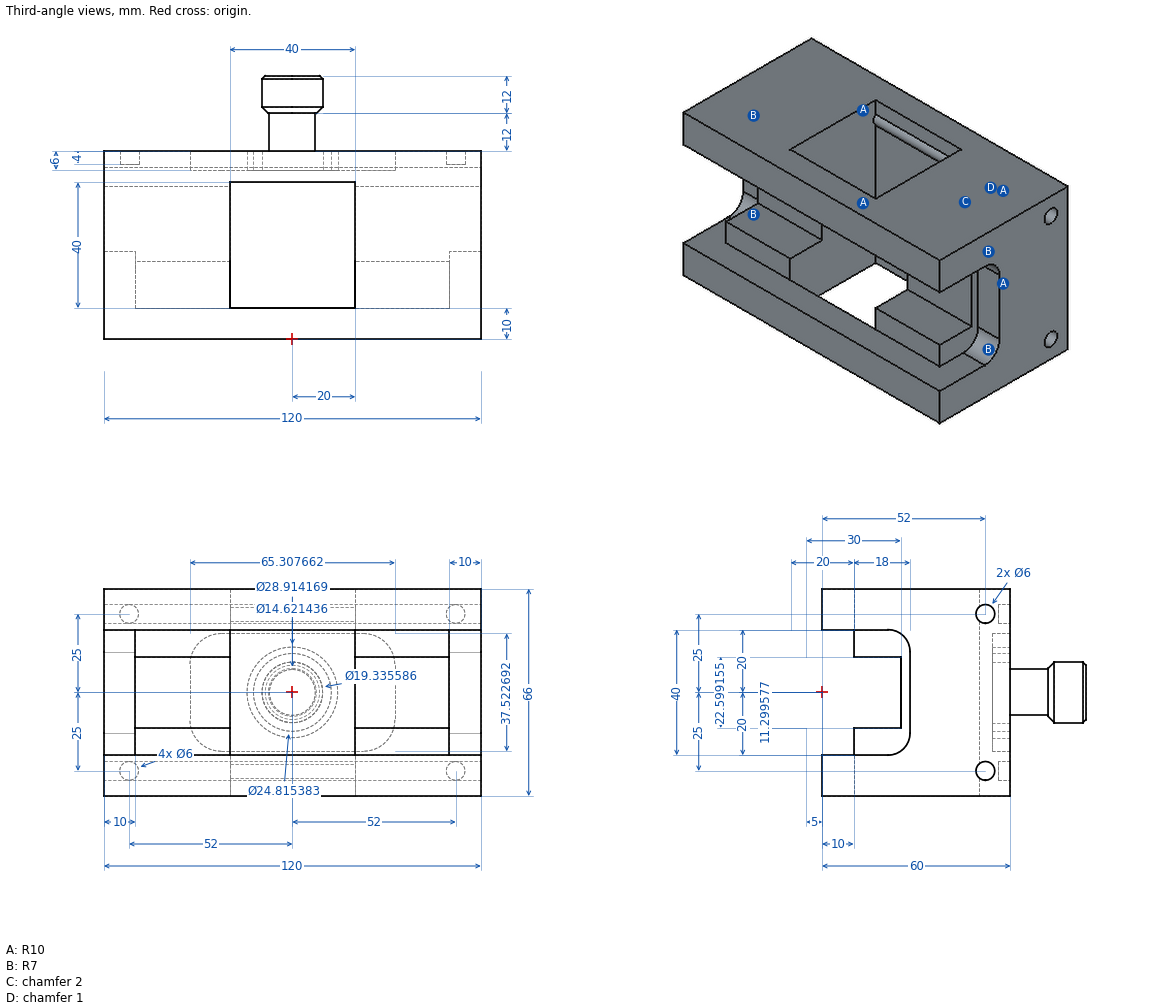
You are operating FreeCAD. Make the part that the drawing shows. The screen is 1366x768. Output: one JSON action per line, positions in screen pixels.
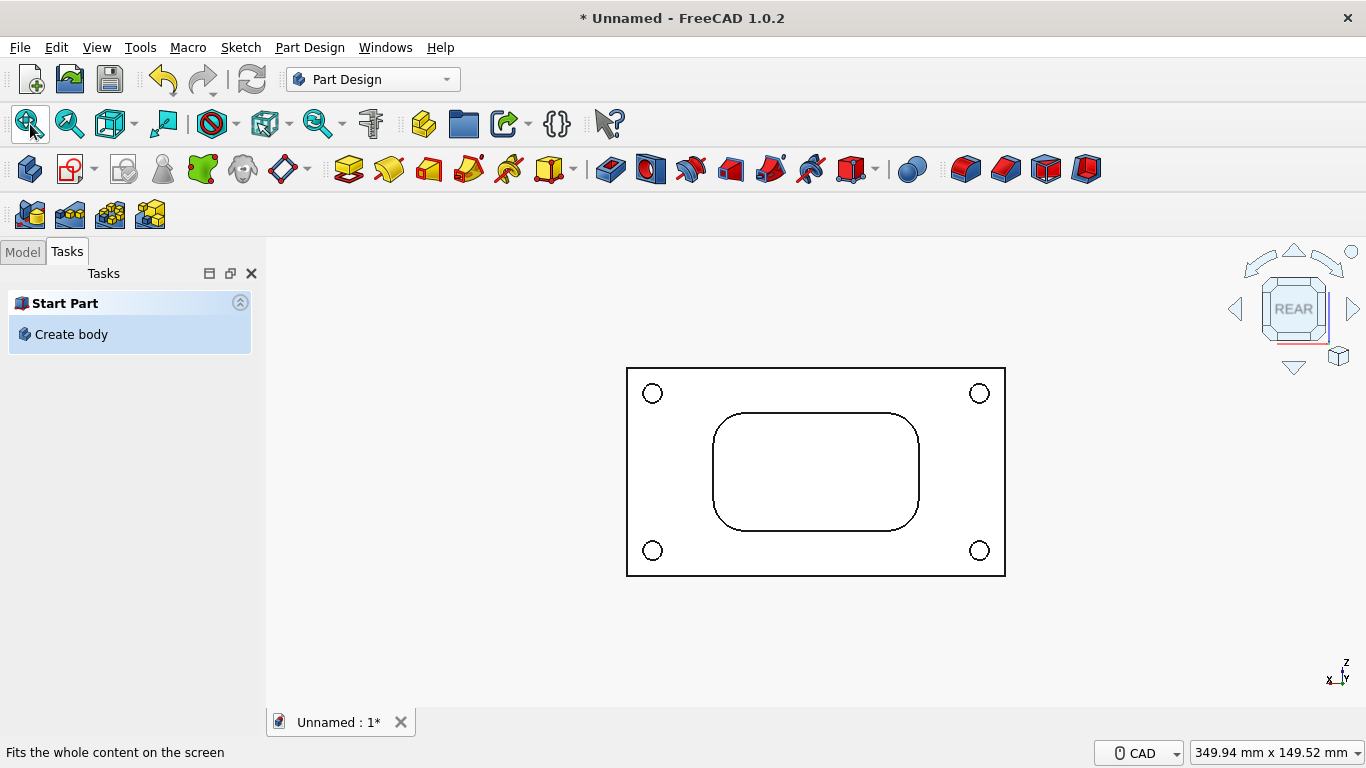
{"action": "left_click", "coordinate": [30, 124]}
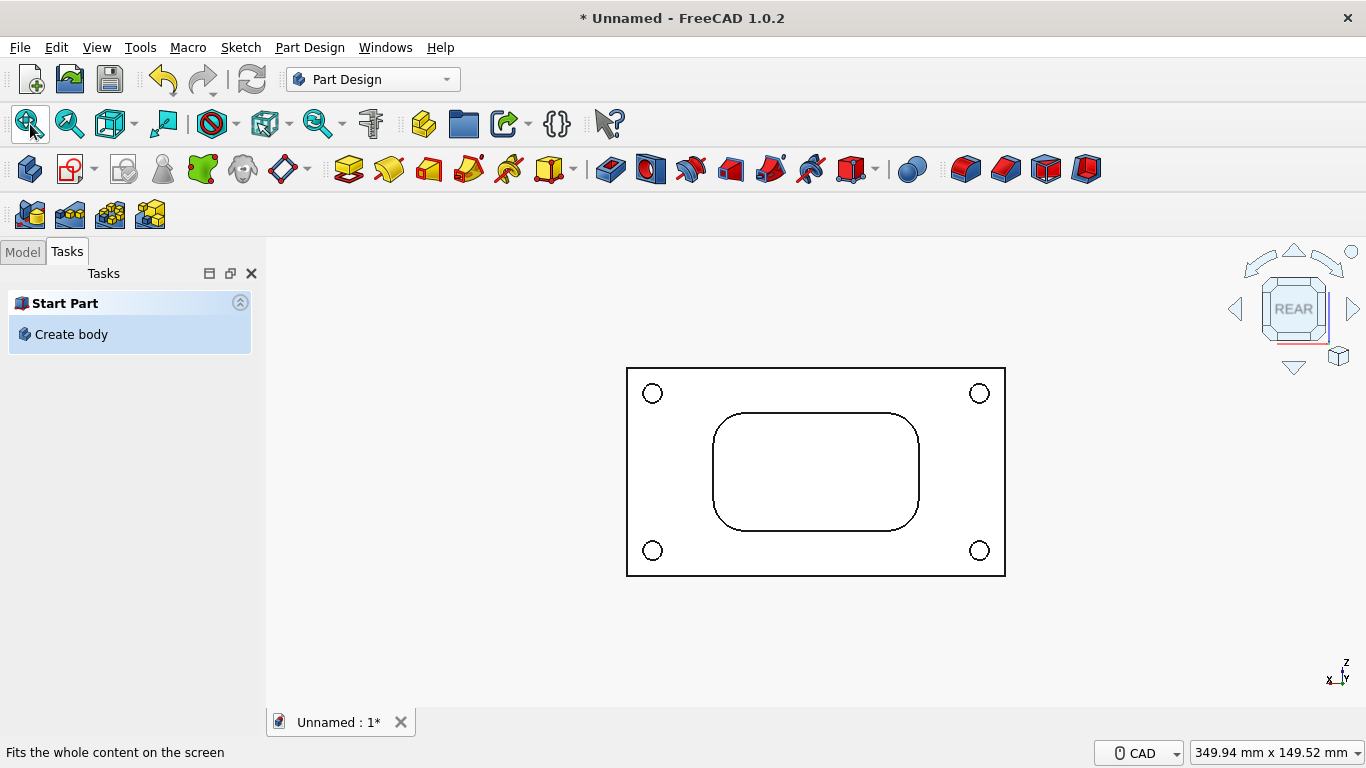
{"action": "key", "text": "6"}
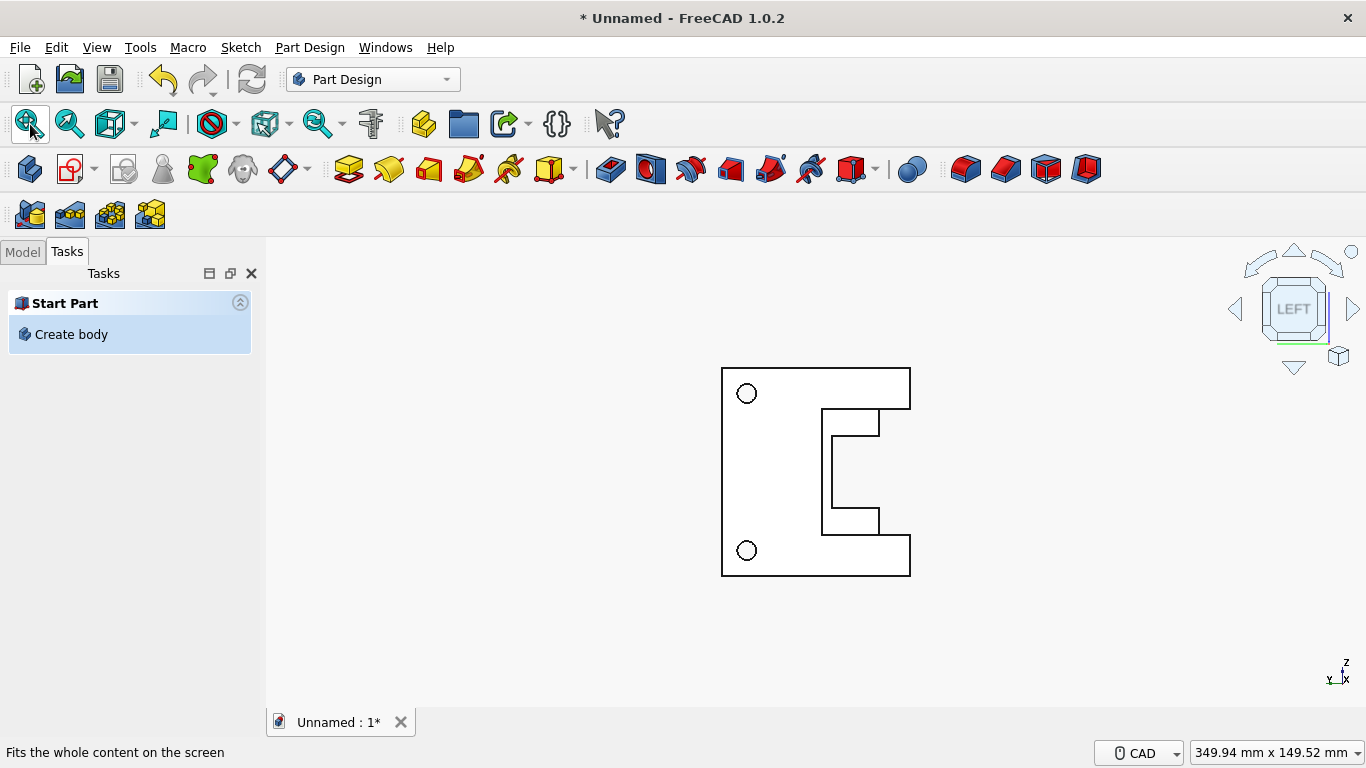
{"action": "left_click", "coordinate": [30, 124]}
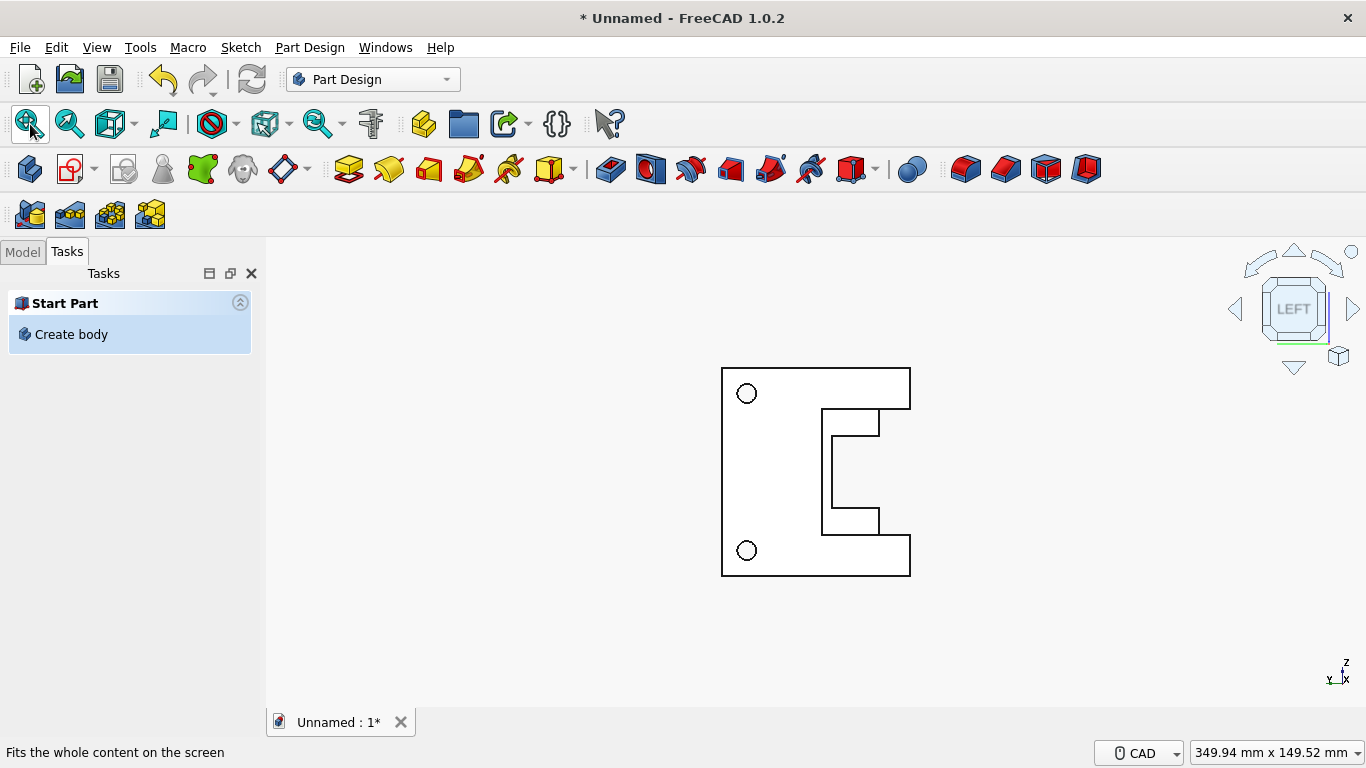
{"action": "key", "text": "v 3"}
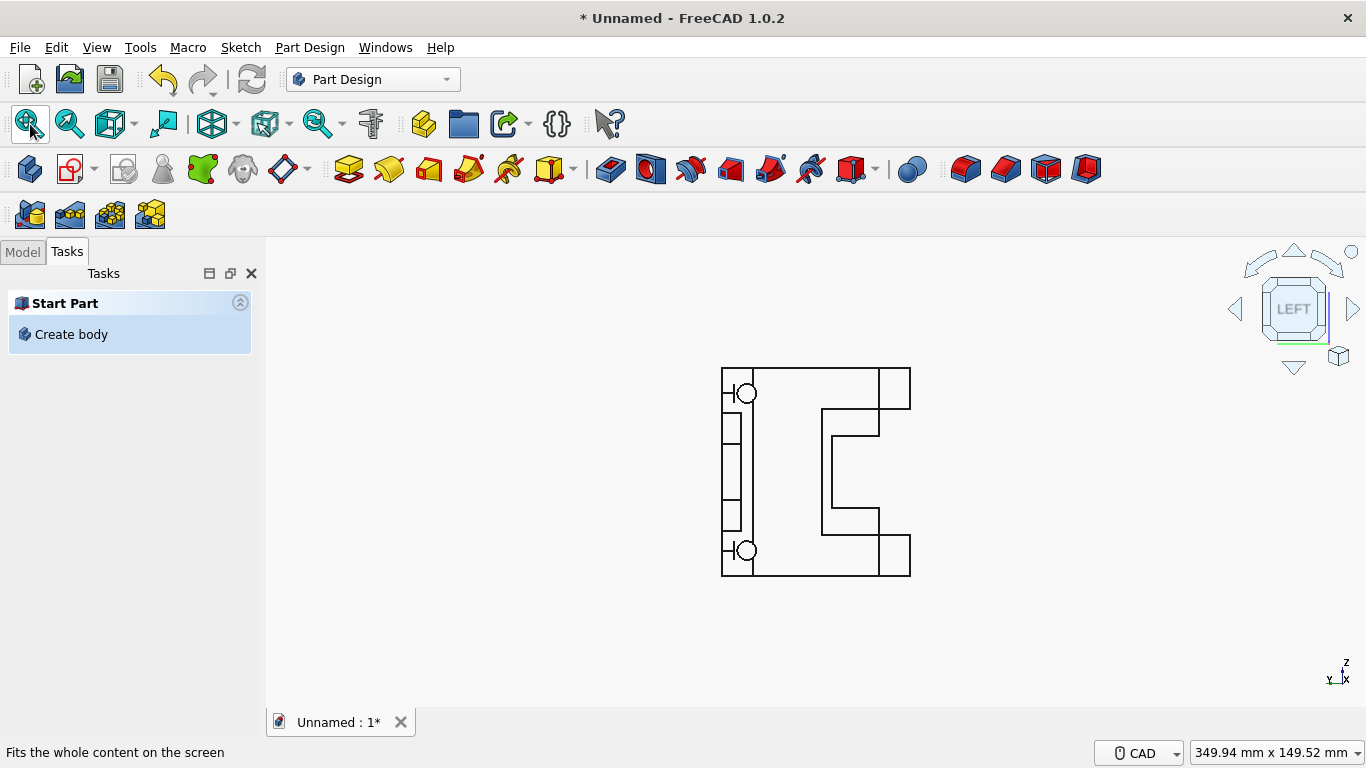
{"action": "key", "text": "0"}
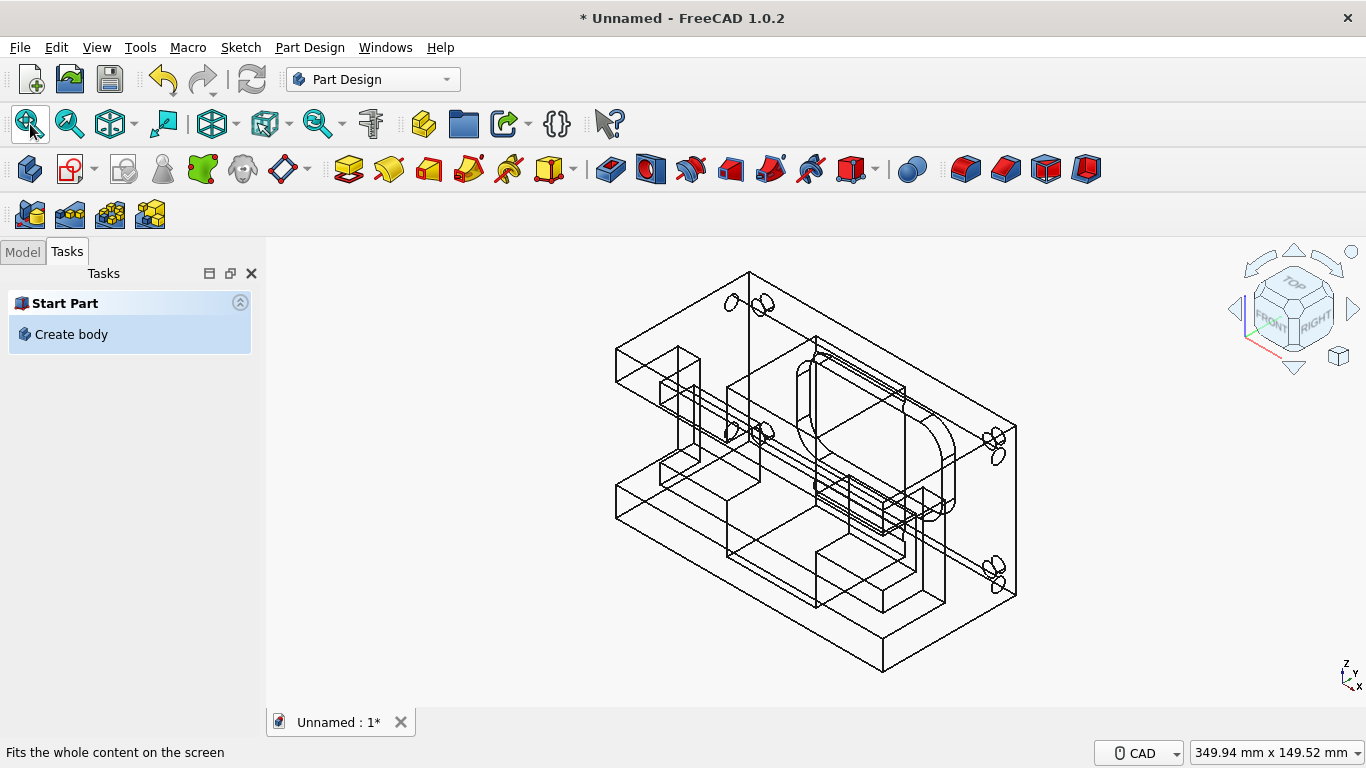
{"action": "left_click", "coordinate": [934, 493]}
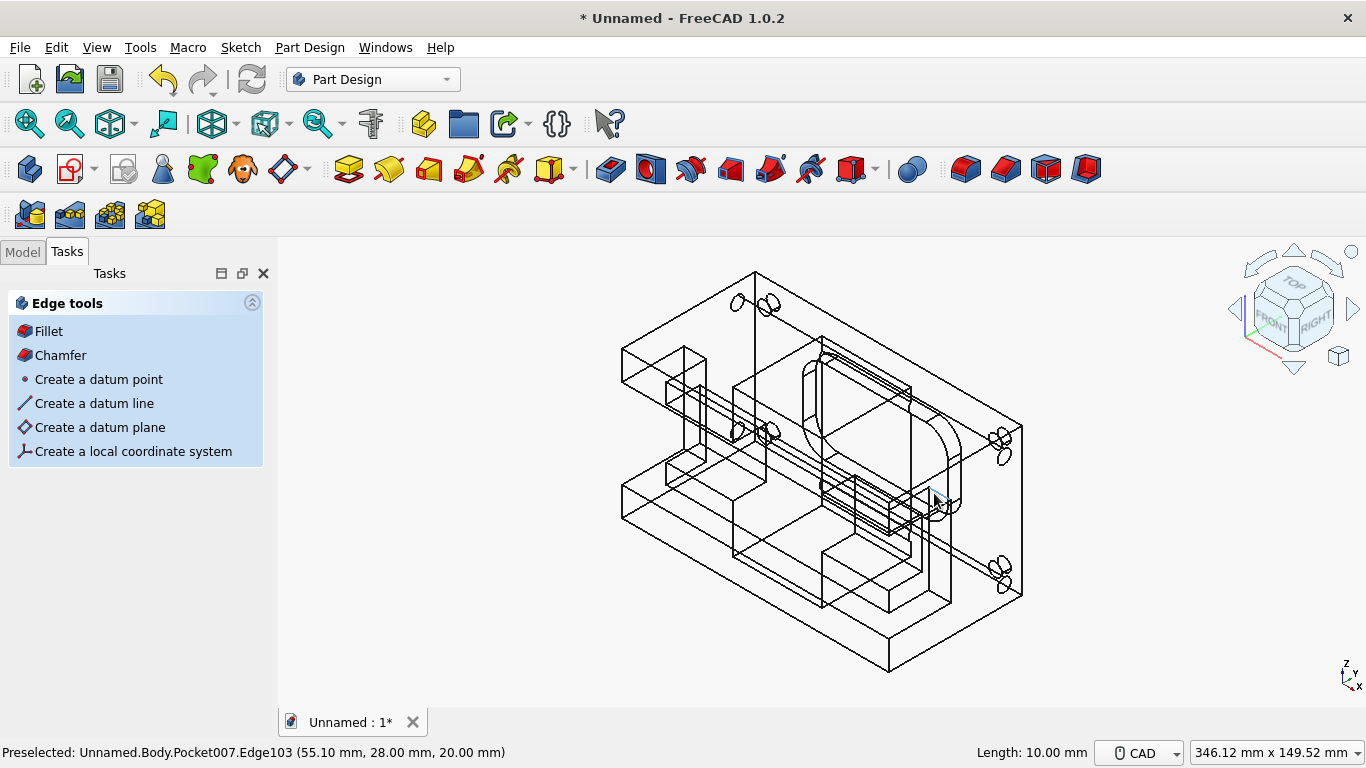
{"action": "left_click", "coordinate": [940, 595], "text": "ctrl"}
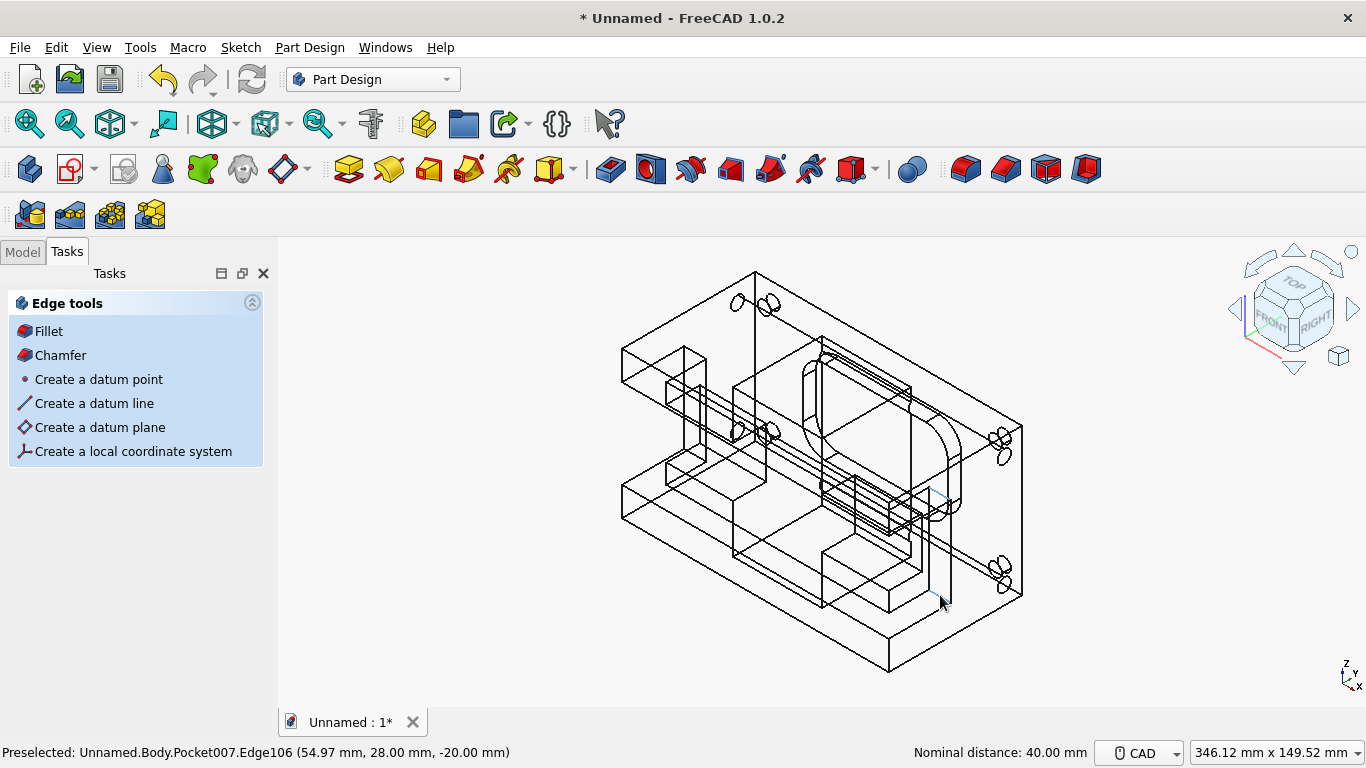
{"action": "left_click", "coordinate": [695, 454], "text": "ctrl"}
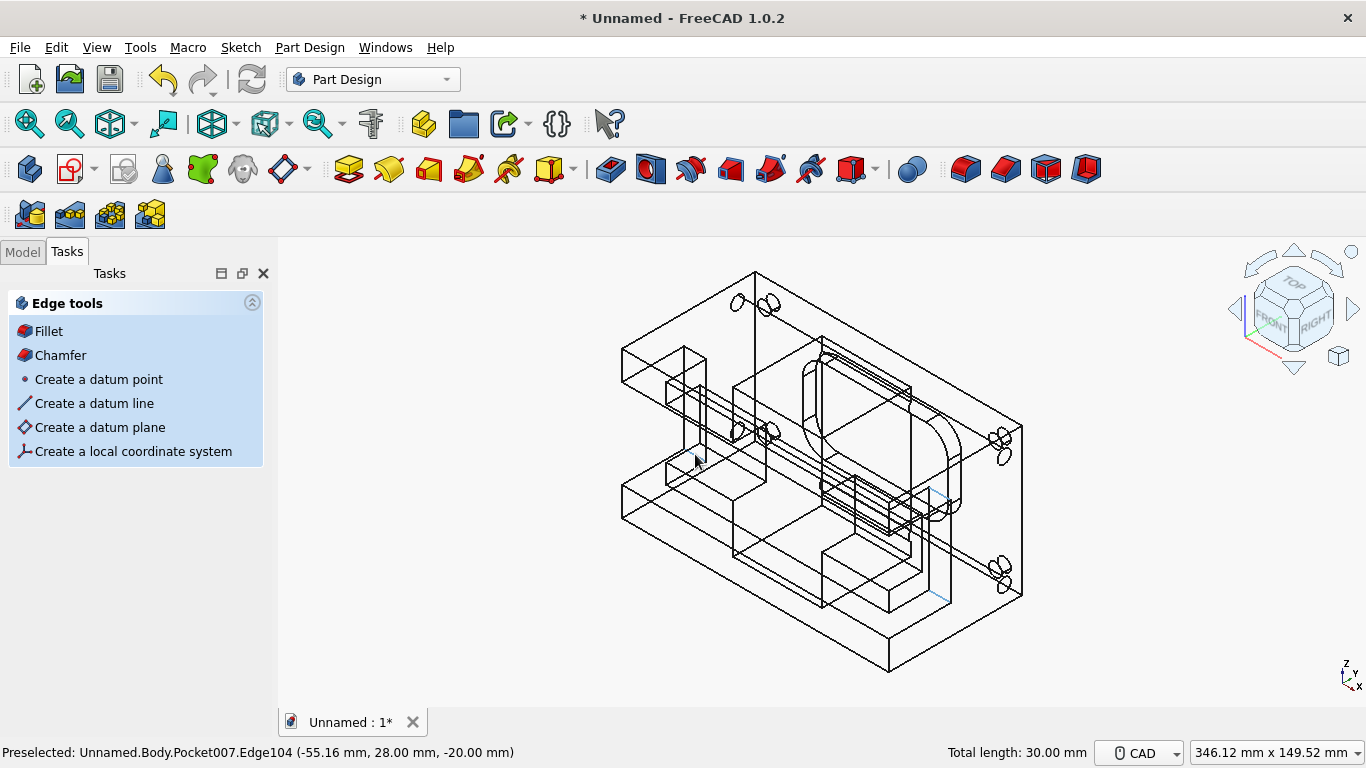
{"action": "left_click", "coordinate": [695, 352], "text": "ctrl"}